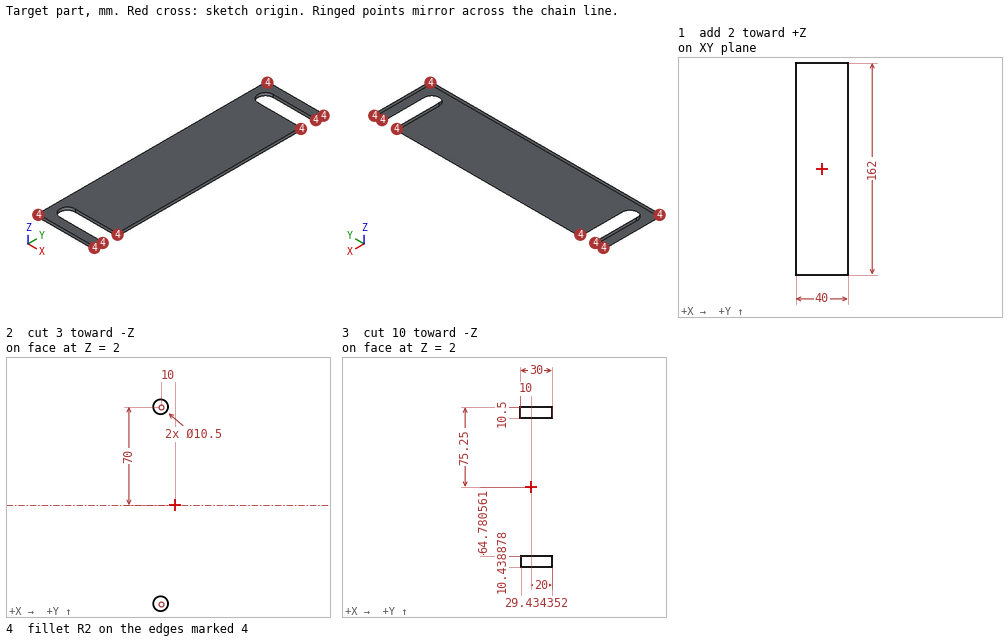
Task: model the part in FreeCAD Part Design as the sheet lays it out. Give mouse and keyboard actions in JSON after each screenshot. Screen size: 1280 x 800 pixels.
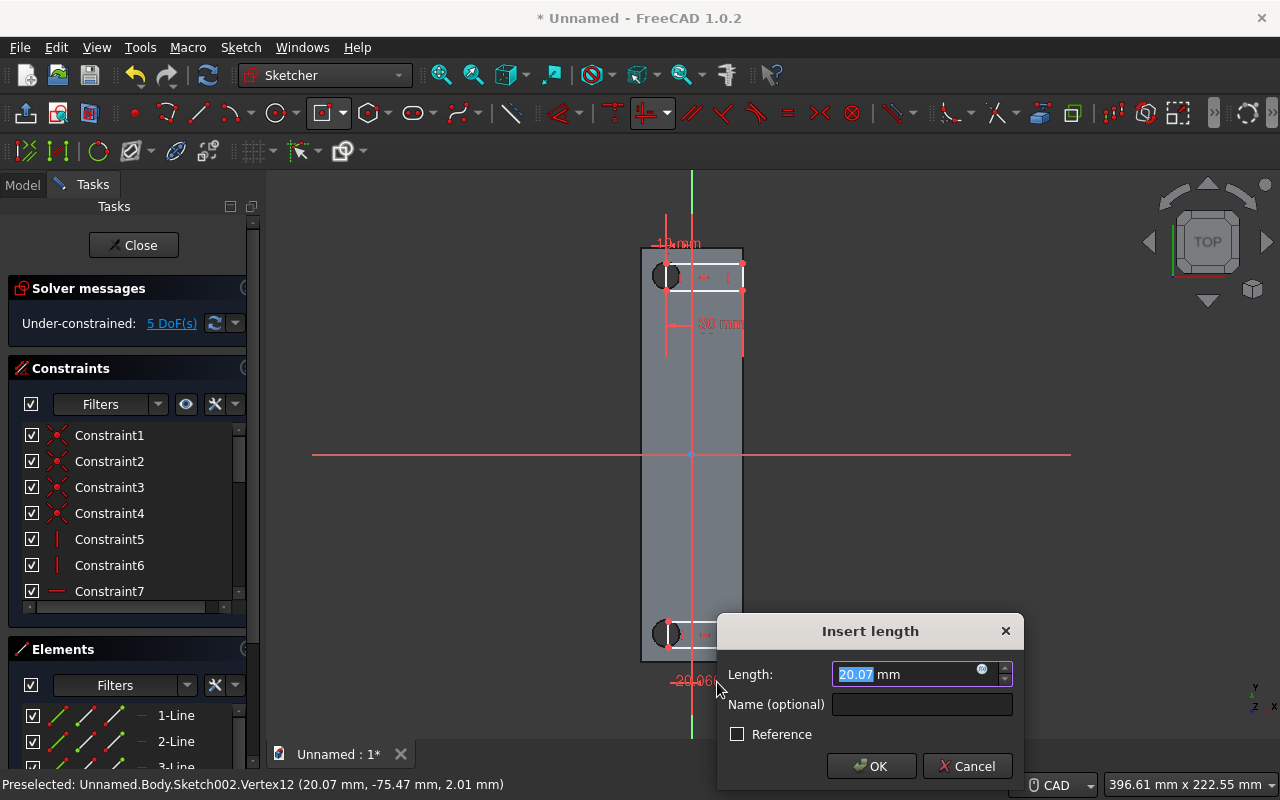
{"action": "type", "text": "20"}
{"action": "key", "text": "Return"}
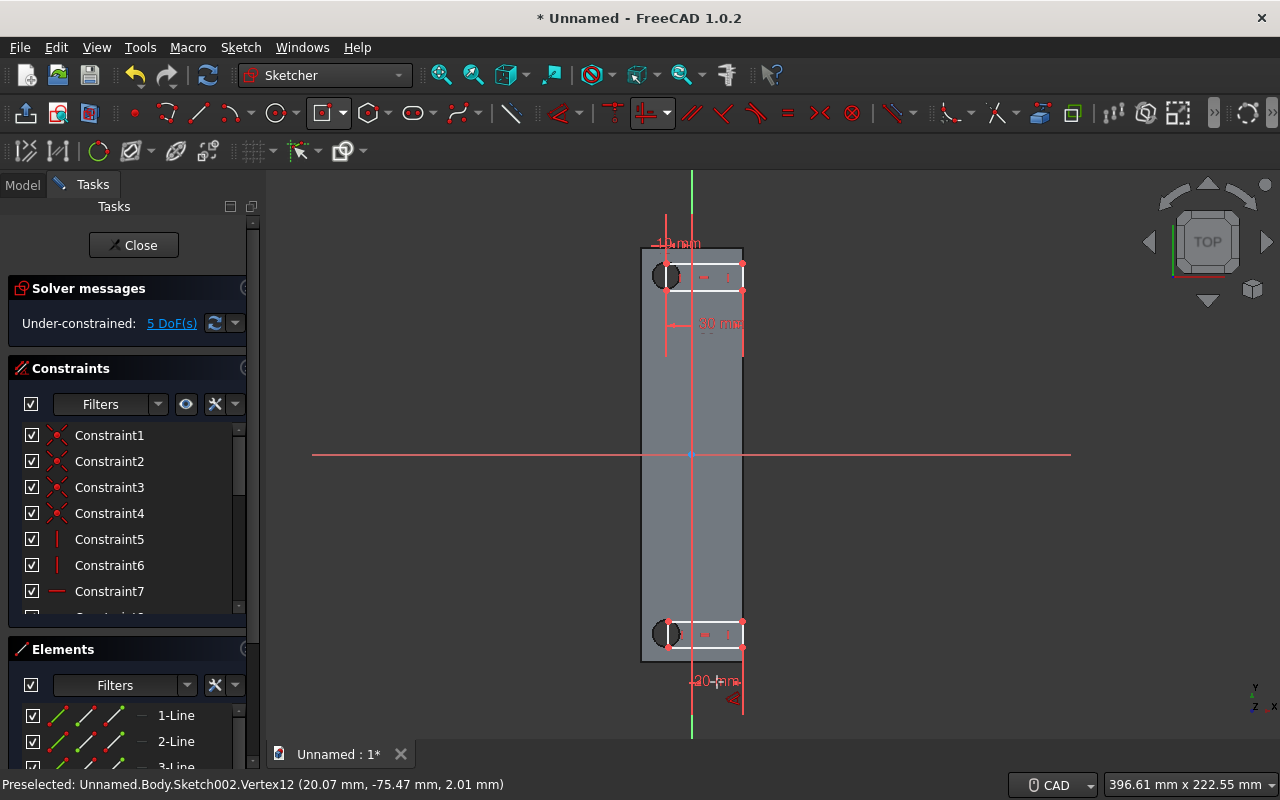
{"action": "scroll", "coordinate": [666, 274], "scroll_direction": "up", "scroll_amount": 2}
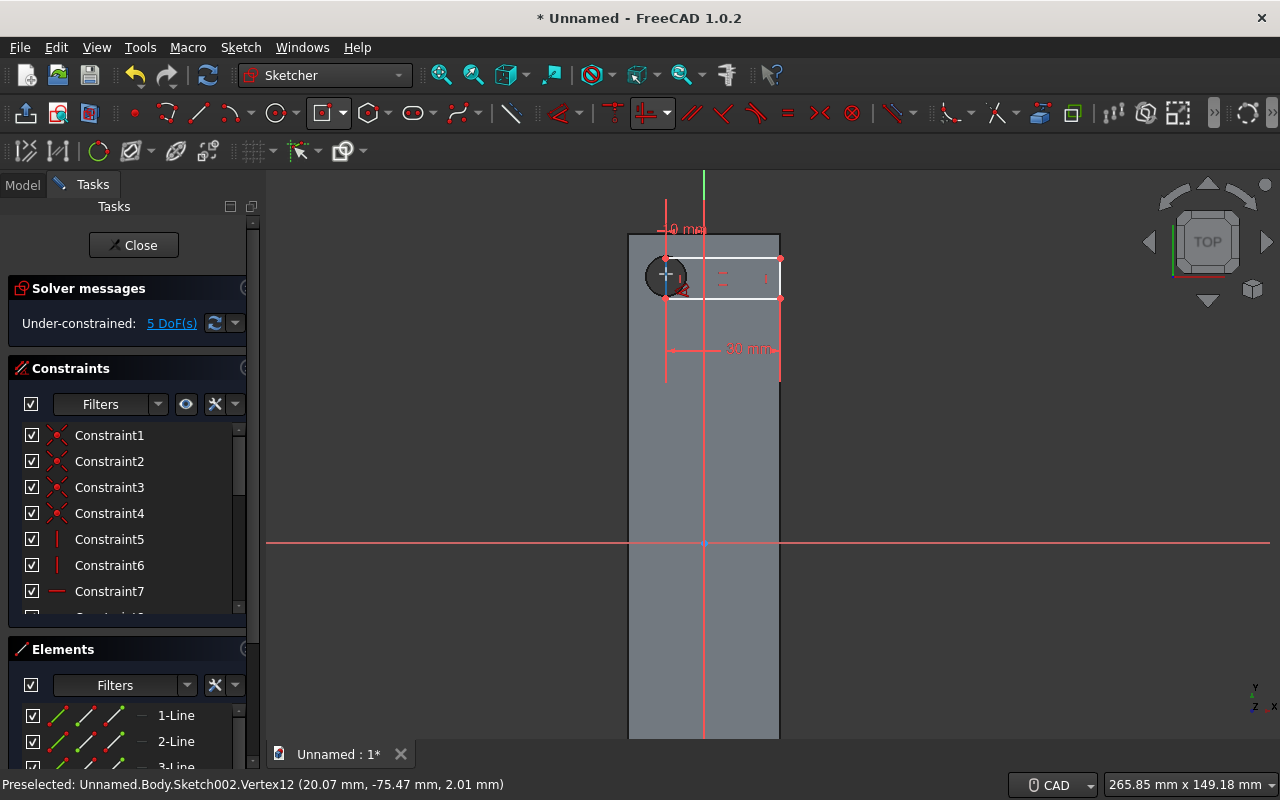
{"action": "left_click", "coordinate": [666, 274]}
{"action": "left_click", "coordinate": [632, 278]}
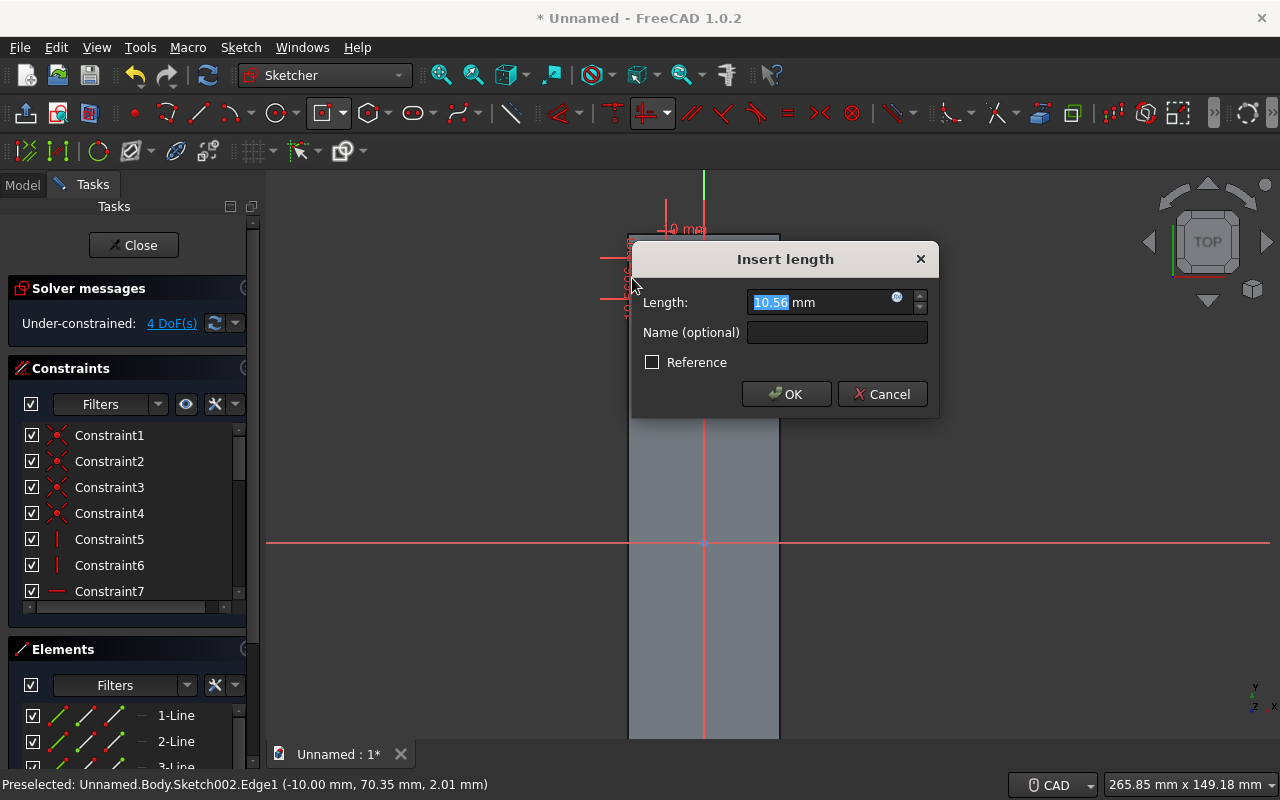
{"action": "type", "text": "10.5"}
{"action": "key", "text": "Return"}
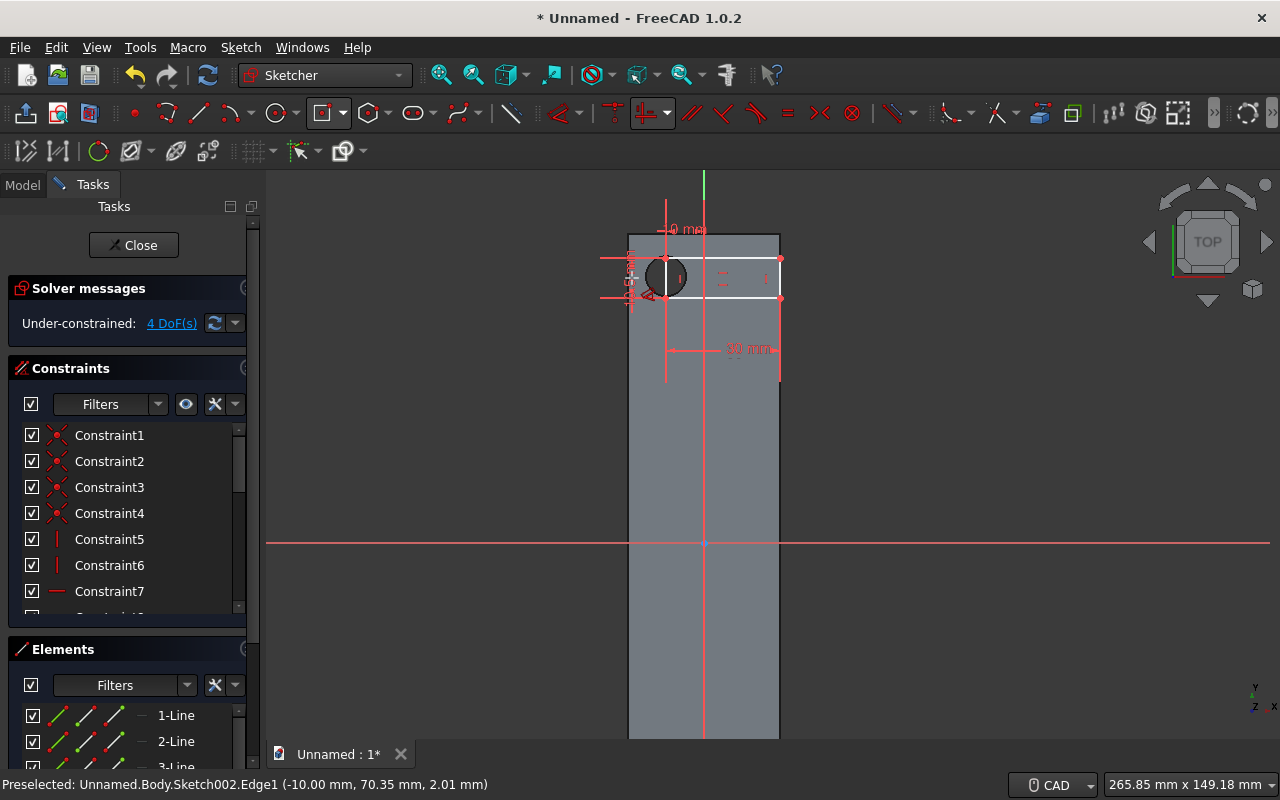
{"action": "left_click", "coordinate": [666, 258]}
{"action": "left_click", "coordinate": [632, 401]}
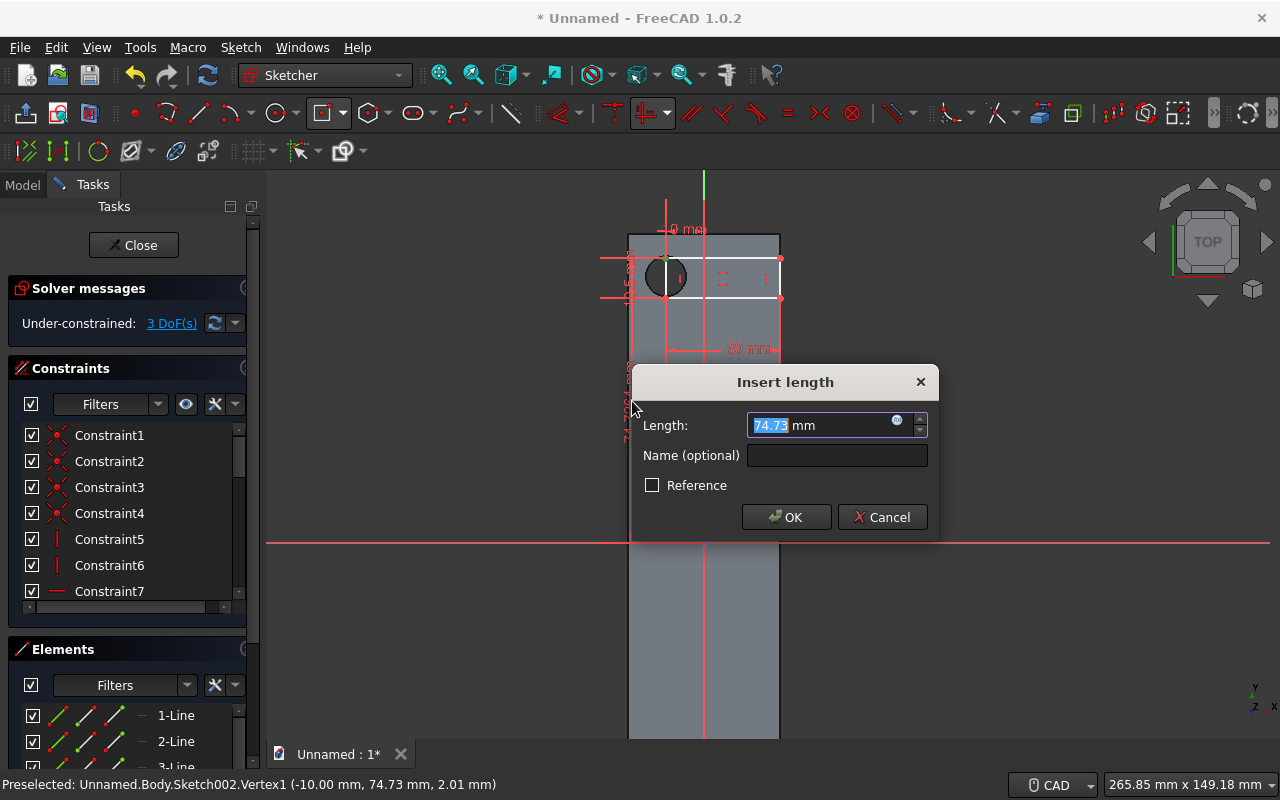
{"action": "type", "text": "75.25"}
{"action": "key", "text": "Return"}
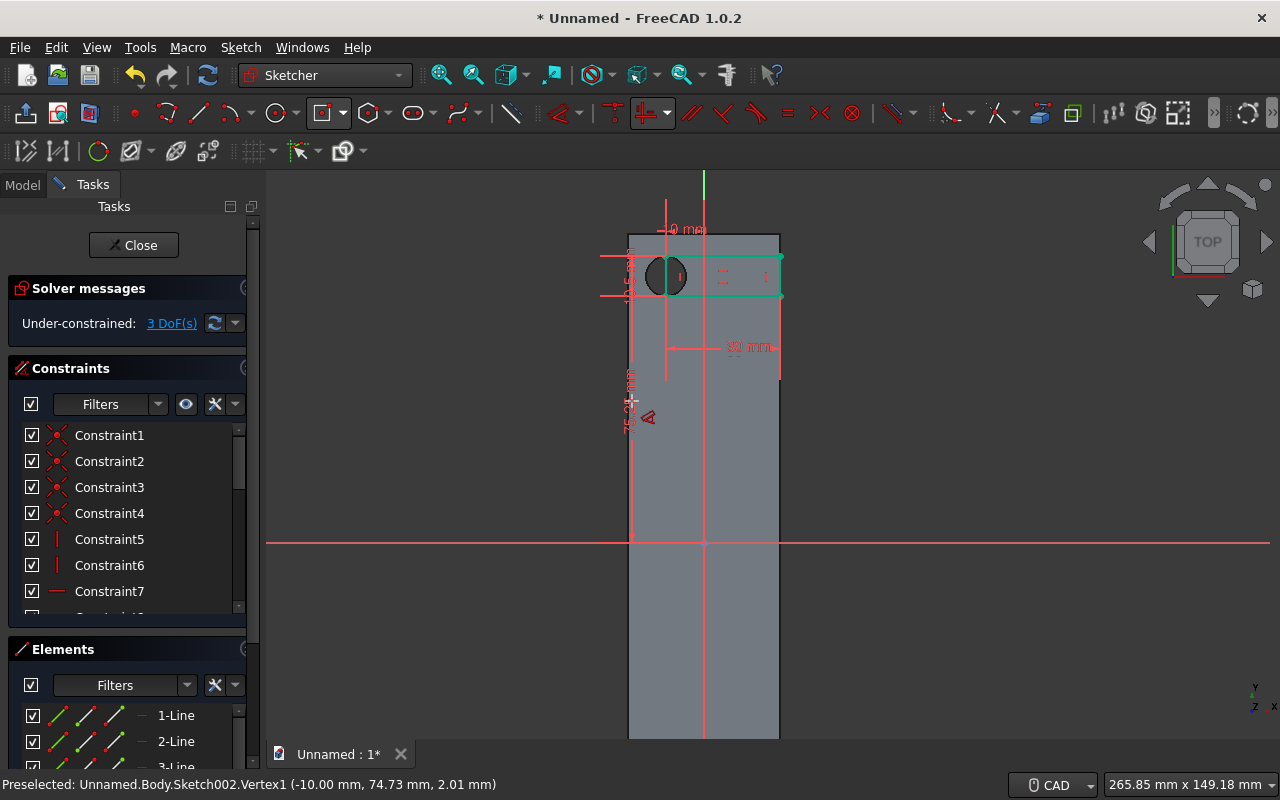
{"action": "scroll", "coordinate": [666, 274], "scroll_direction": "down", "scroll_amount": 2}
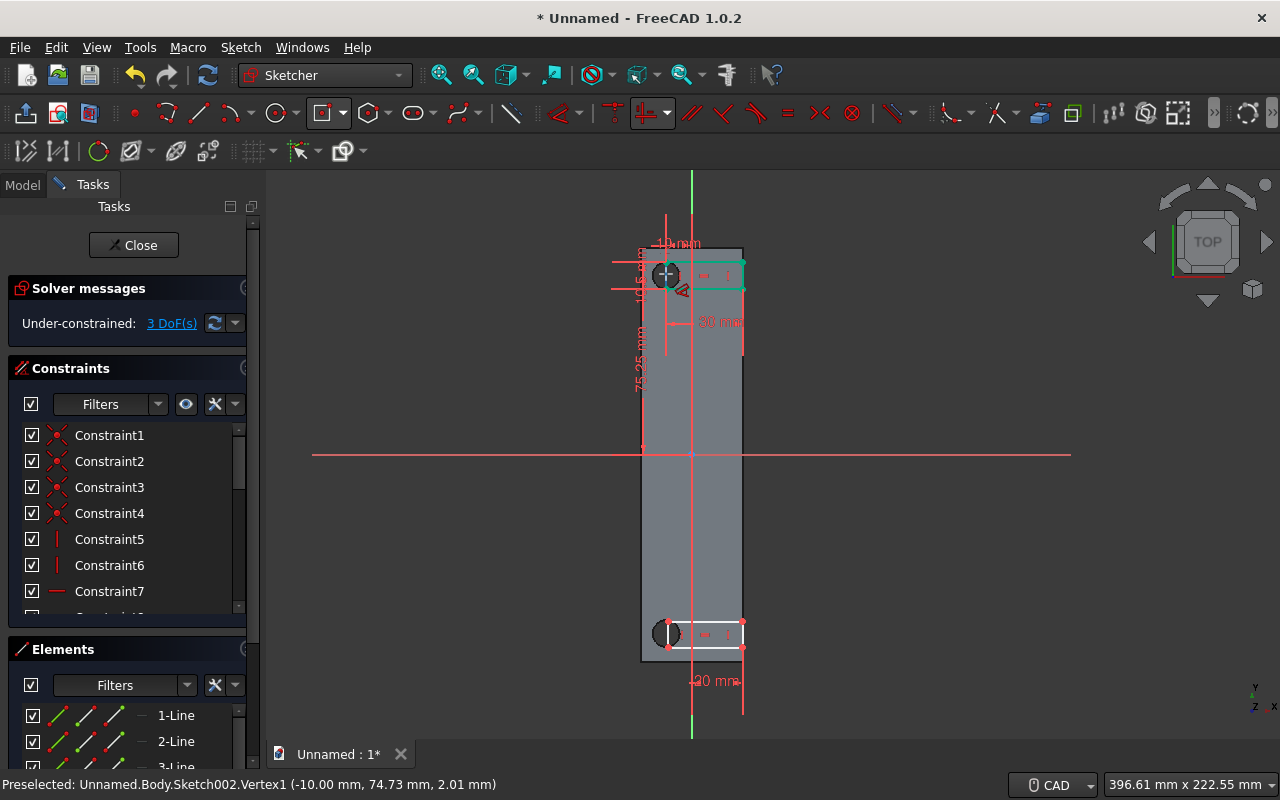
{"action": "scroll", "coordinate": [668, 629], "scroll_direction": "up", "scroll_amount": 3}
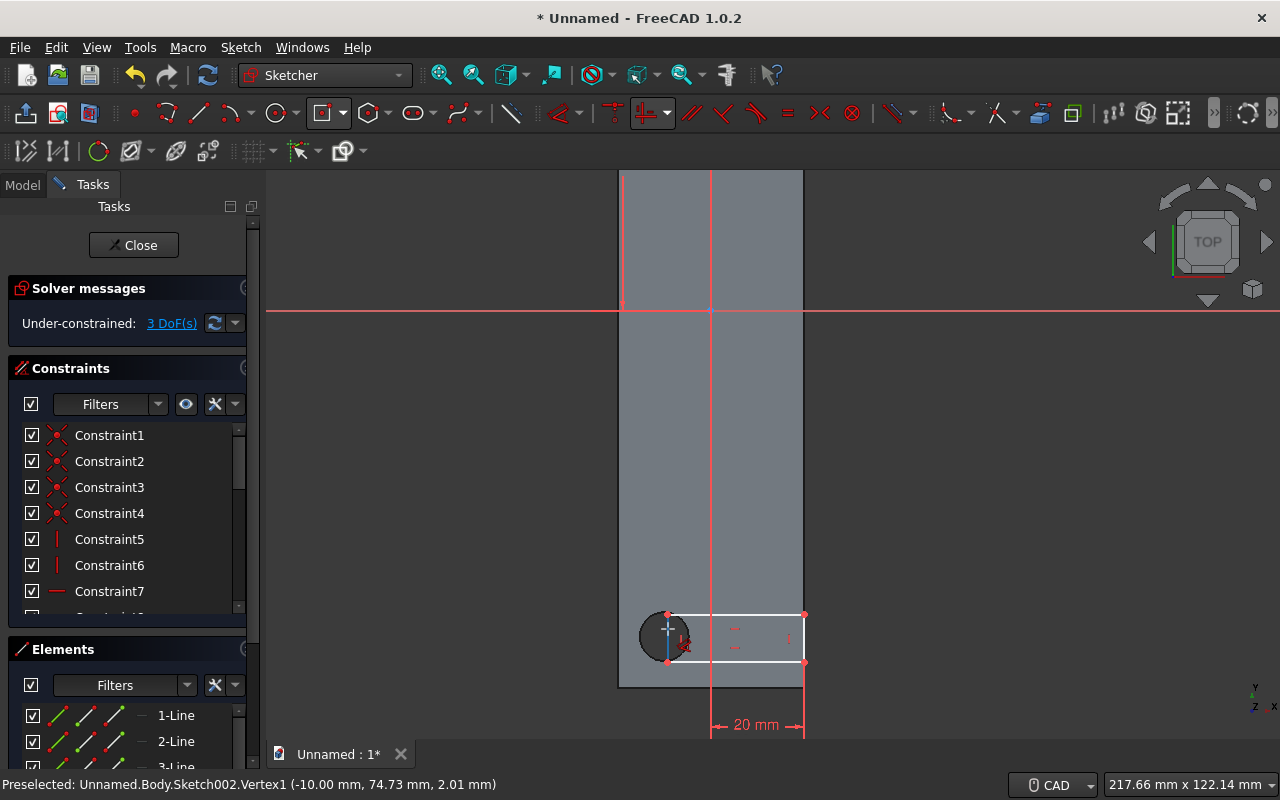
{"action": "left_click", "coordinate": [668, 629]}
{"action": "left_click", "coordinate": [634, 638]}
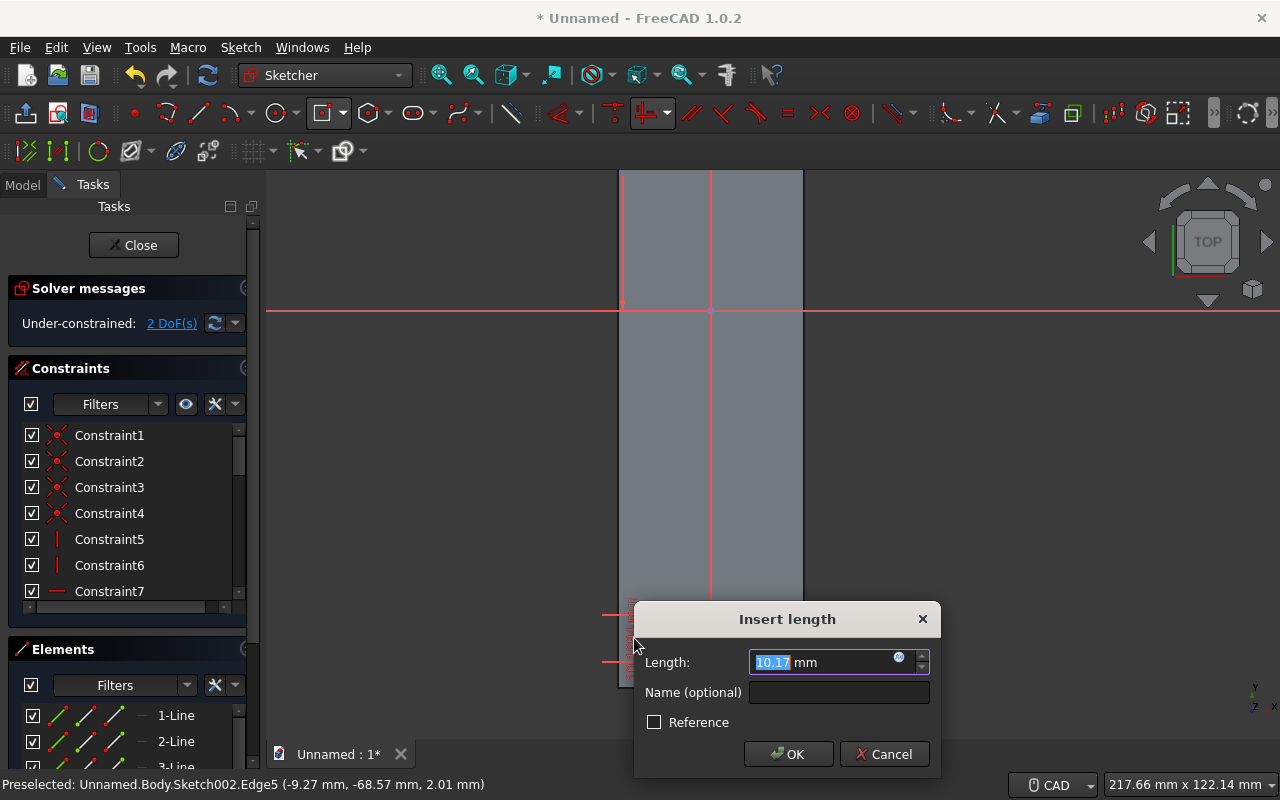
{"action": "type", "text": "10.438878"}
{"action": "key", "text": "Return"}